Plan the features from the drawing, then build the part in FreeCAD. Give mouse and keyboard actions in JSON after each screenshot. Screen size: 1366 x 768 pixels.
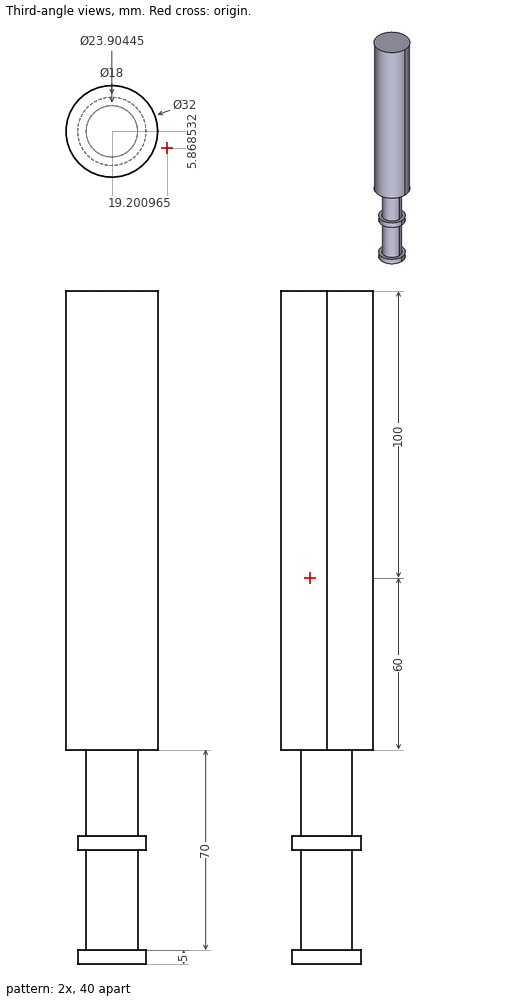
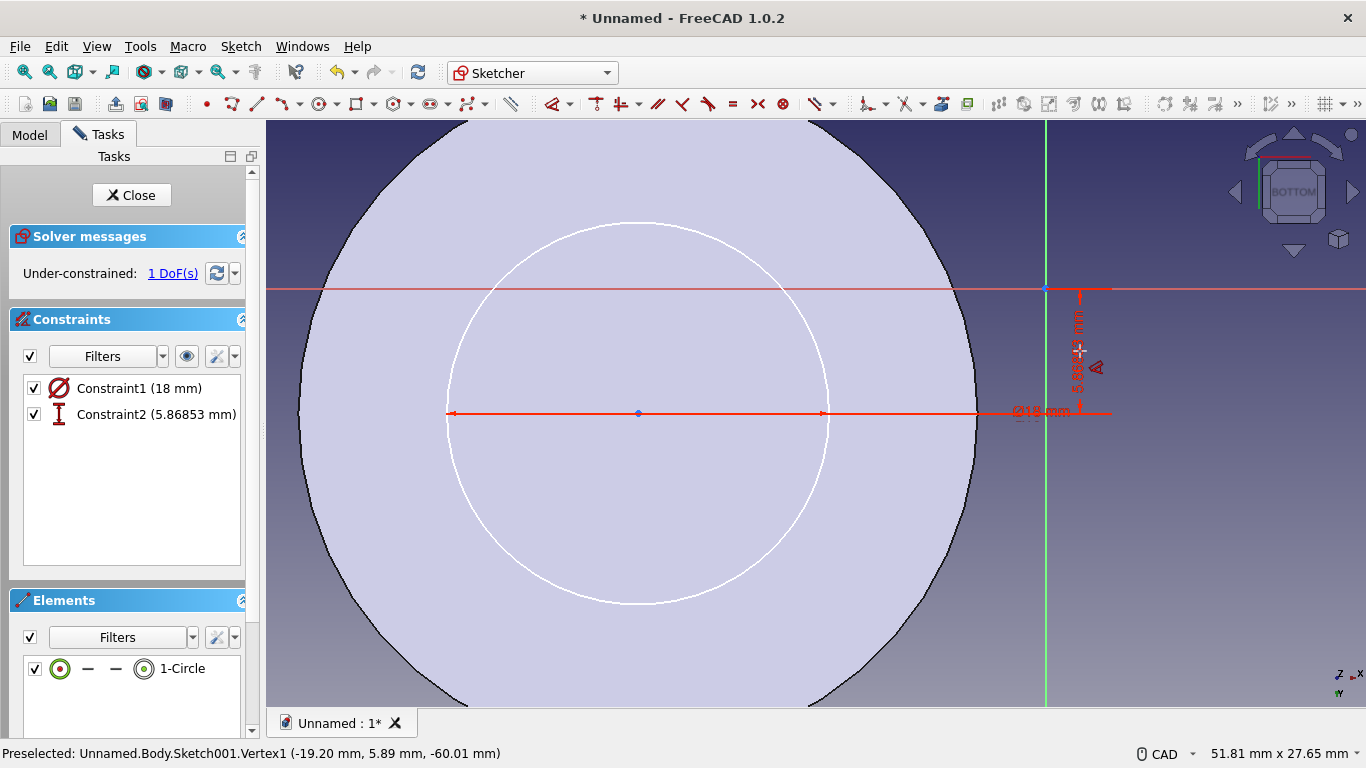
{"action": "left_click", "coordinate": [638, 413]}
{"action": "left_click", "coordinate": [842, 255]}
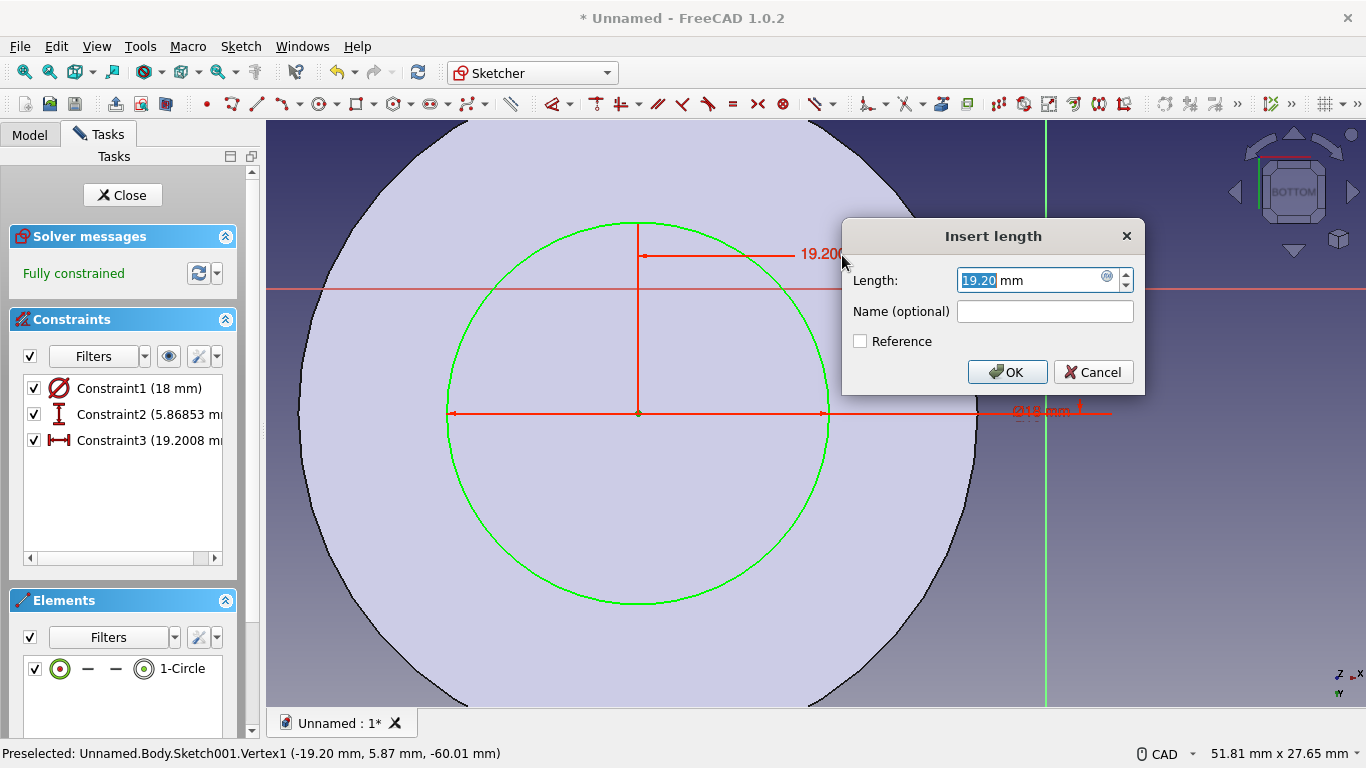
{"action": "type", "text": "19.200965"}
{"action": "key", "text": "Return"}
{"action": "key", "text": "Escape"}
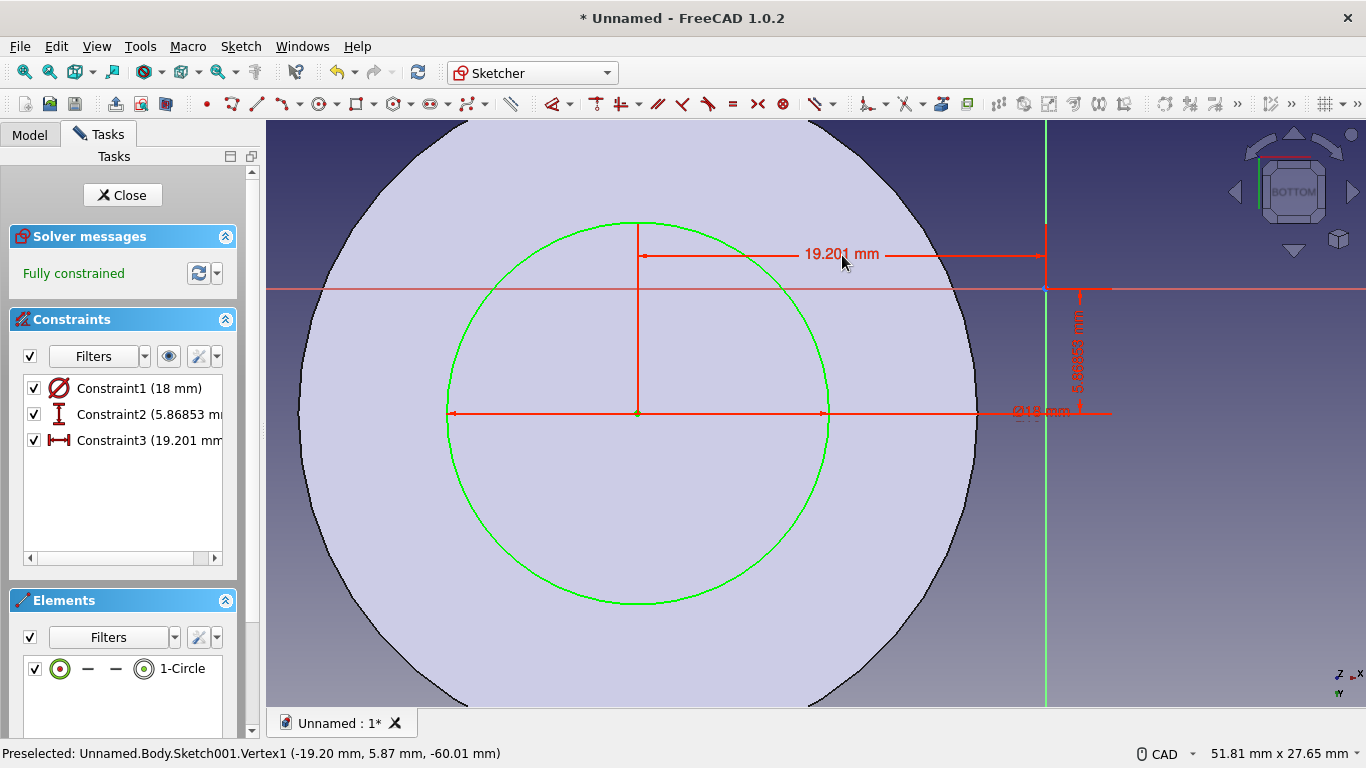
{"action": "left_click", "coordinate": [123, 195]}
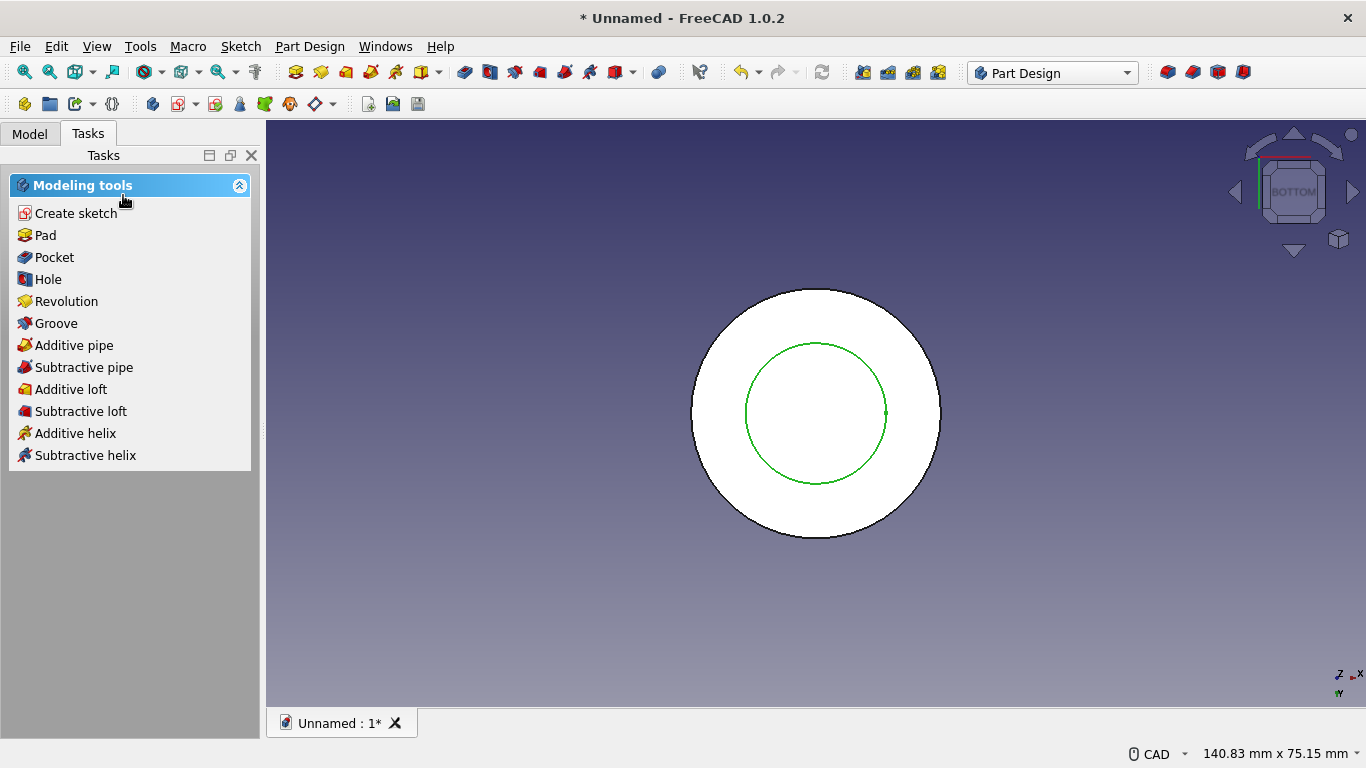
{"action": "left_click", "coordinate": [296, 72]}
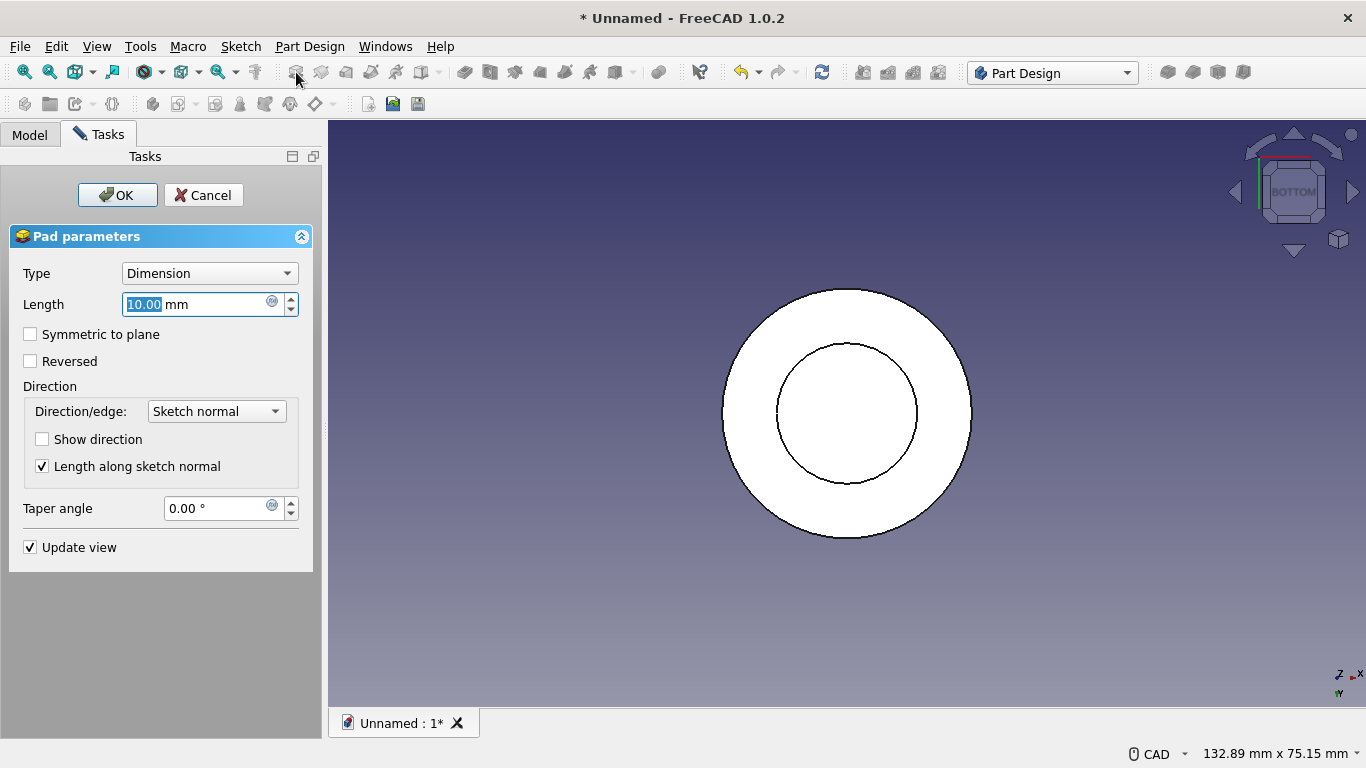
{"action": "type", "text": "70"}
{"action": "key", "text": "Tab"}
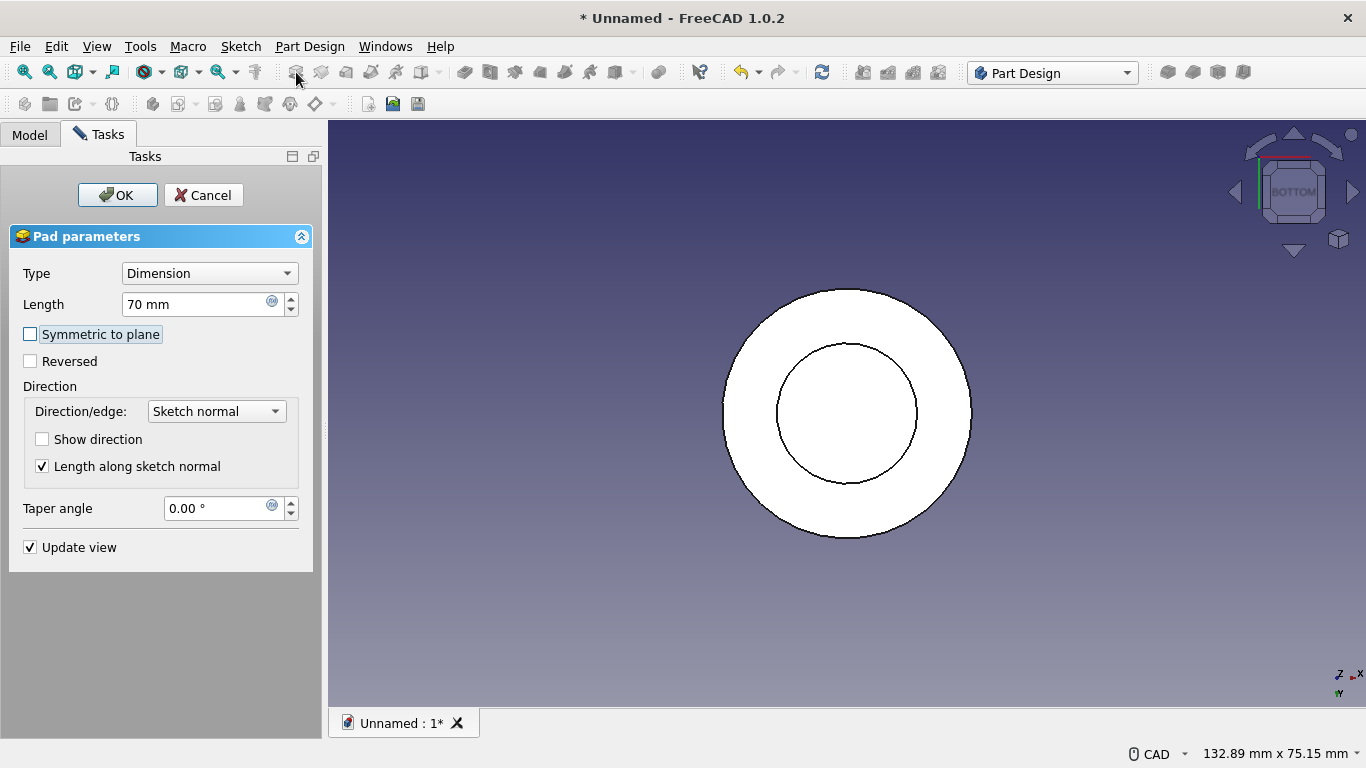
{"action": "left_click", "coordinate": [118, 195]}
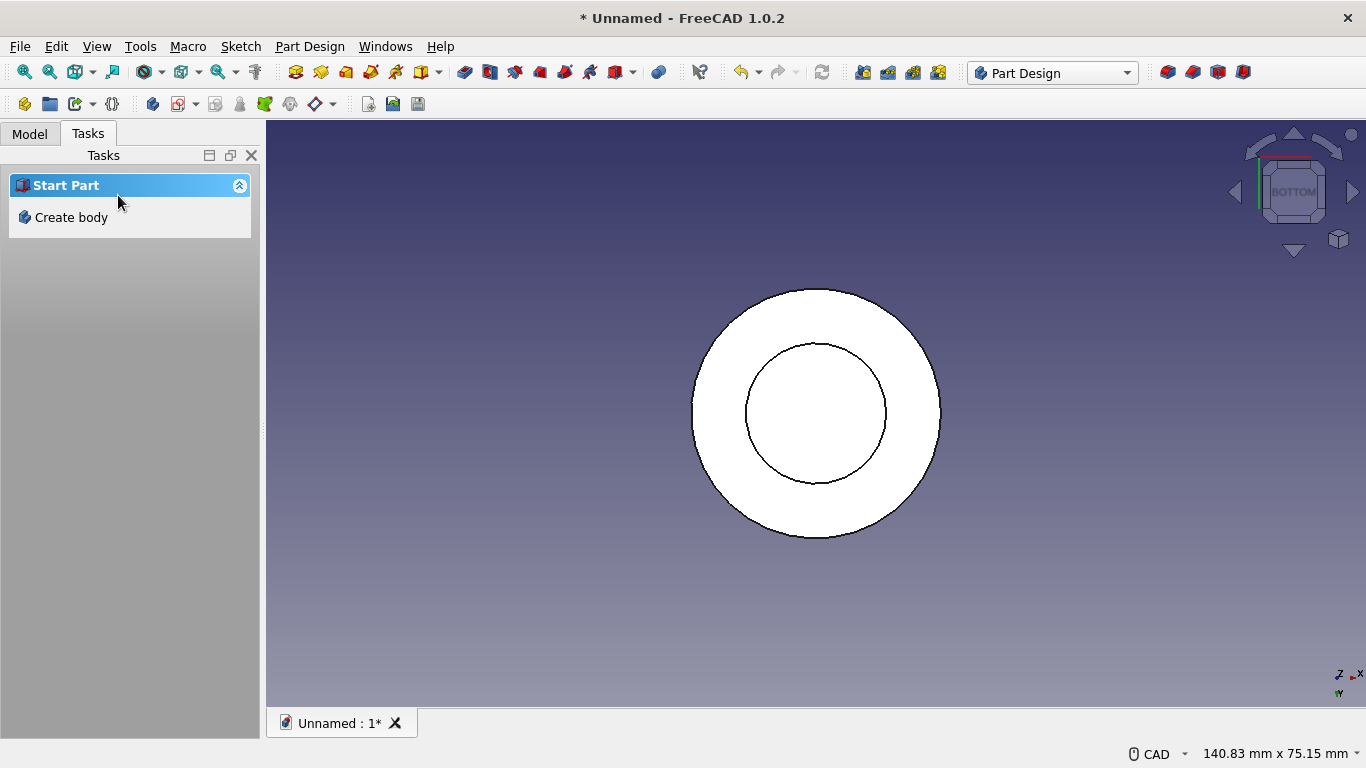
{"action": "key", "text": "v f"}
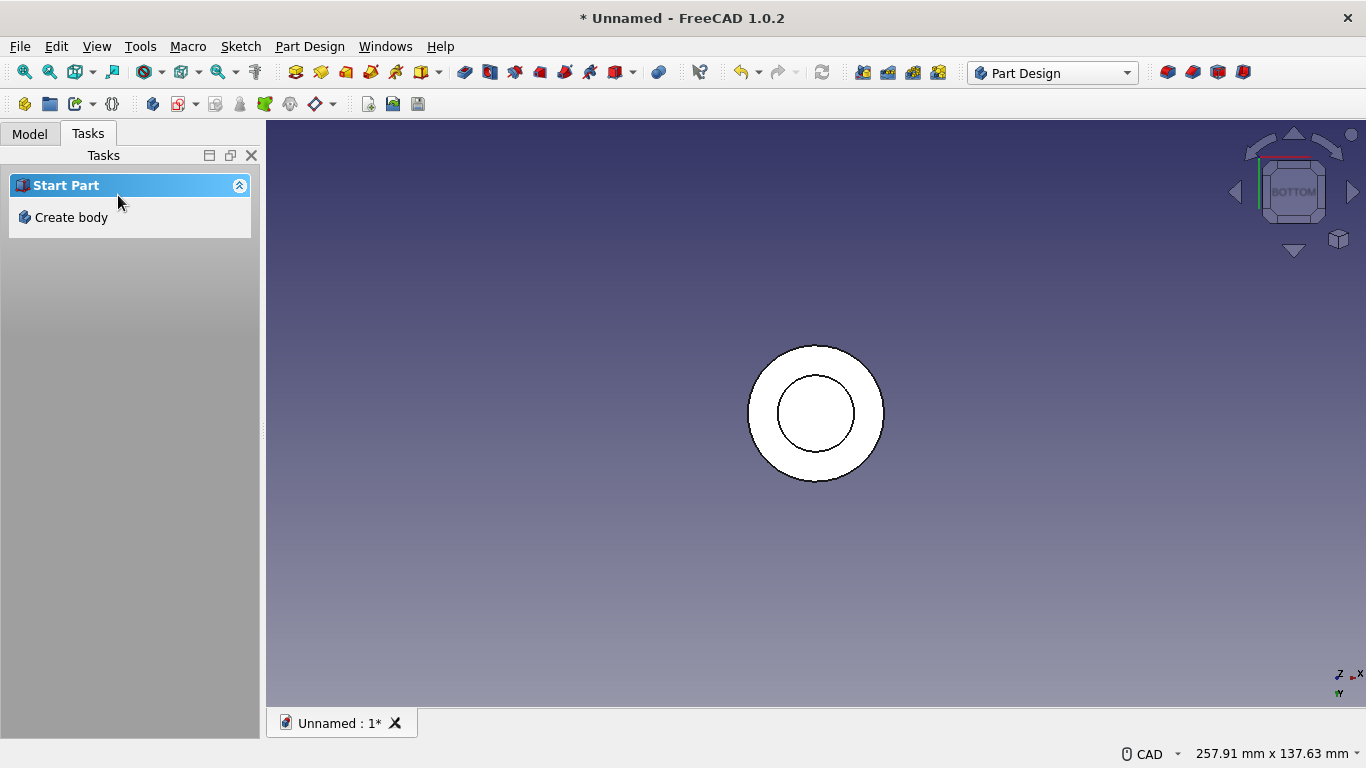
{"action": "left_click", "coordinate": [30, 134]}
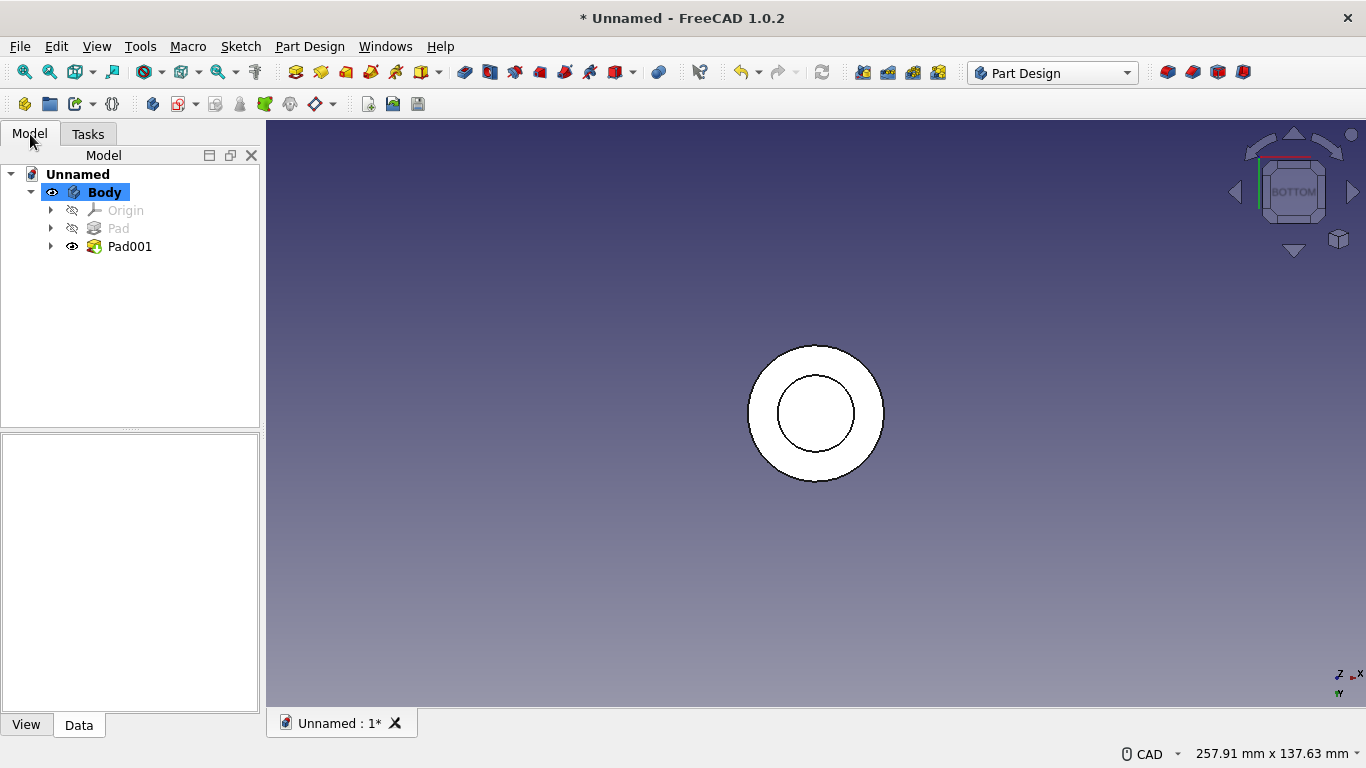
{"action": "left_click", "coordinate": [51, 210]}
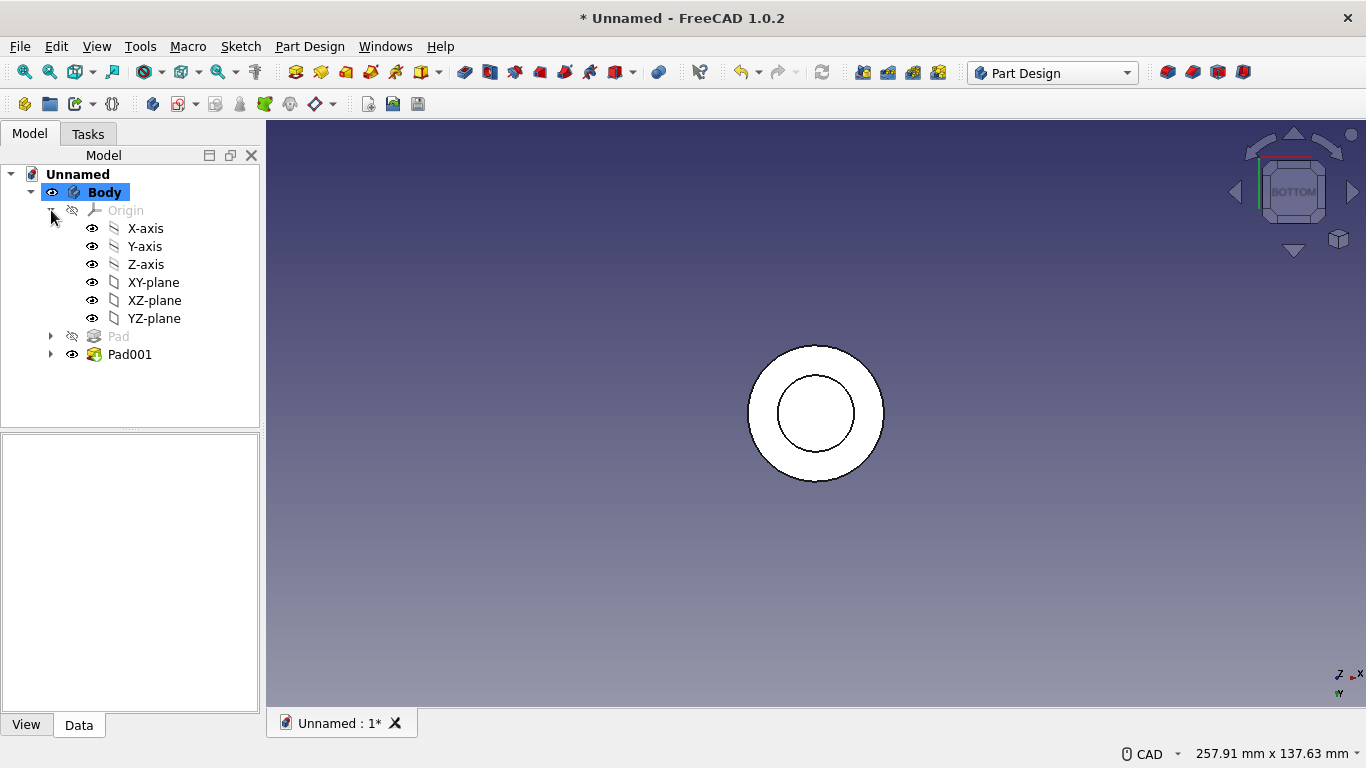
{"action": "left_click", "coordinate": [137, 282]}